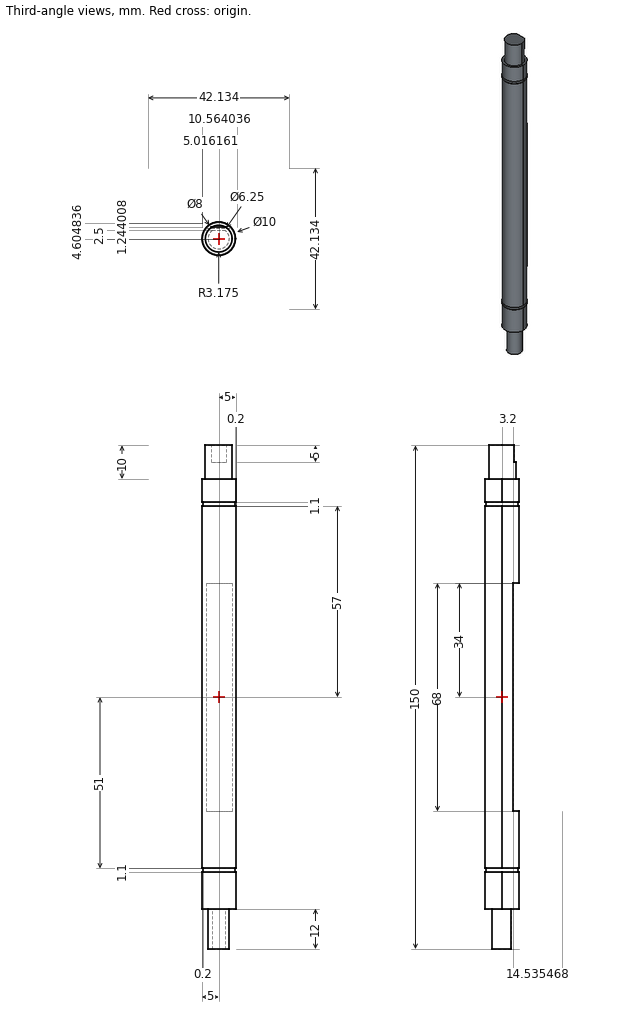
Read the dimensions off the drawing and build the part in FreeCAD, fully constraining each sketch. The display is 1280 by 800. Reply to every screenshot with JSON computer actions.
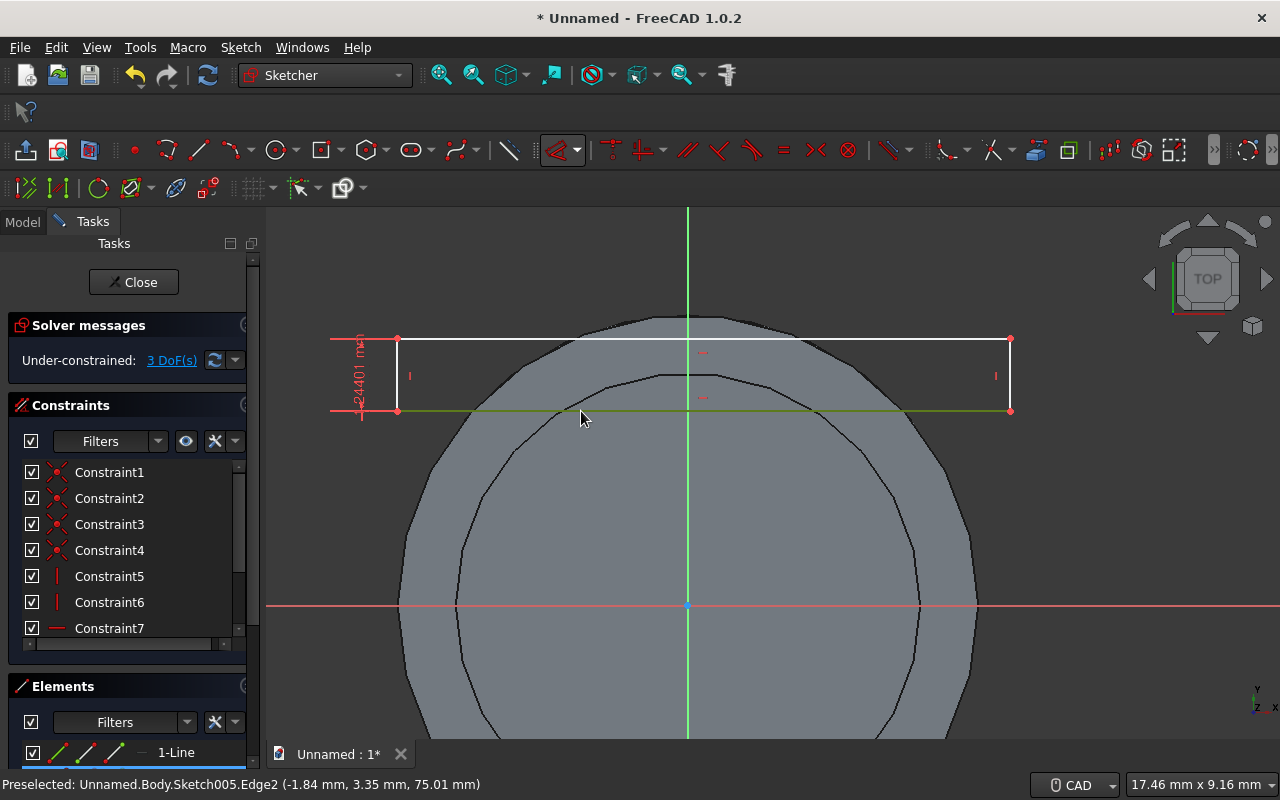
{"action": "key", "text": "l"}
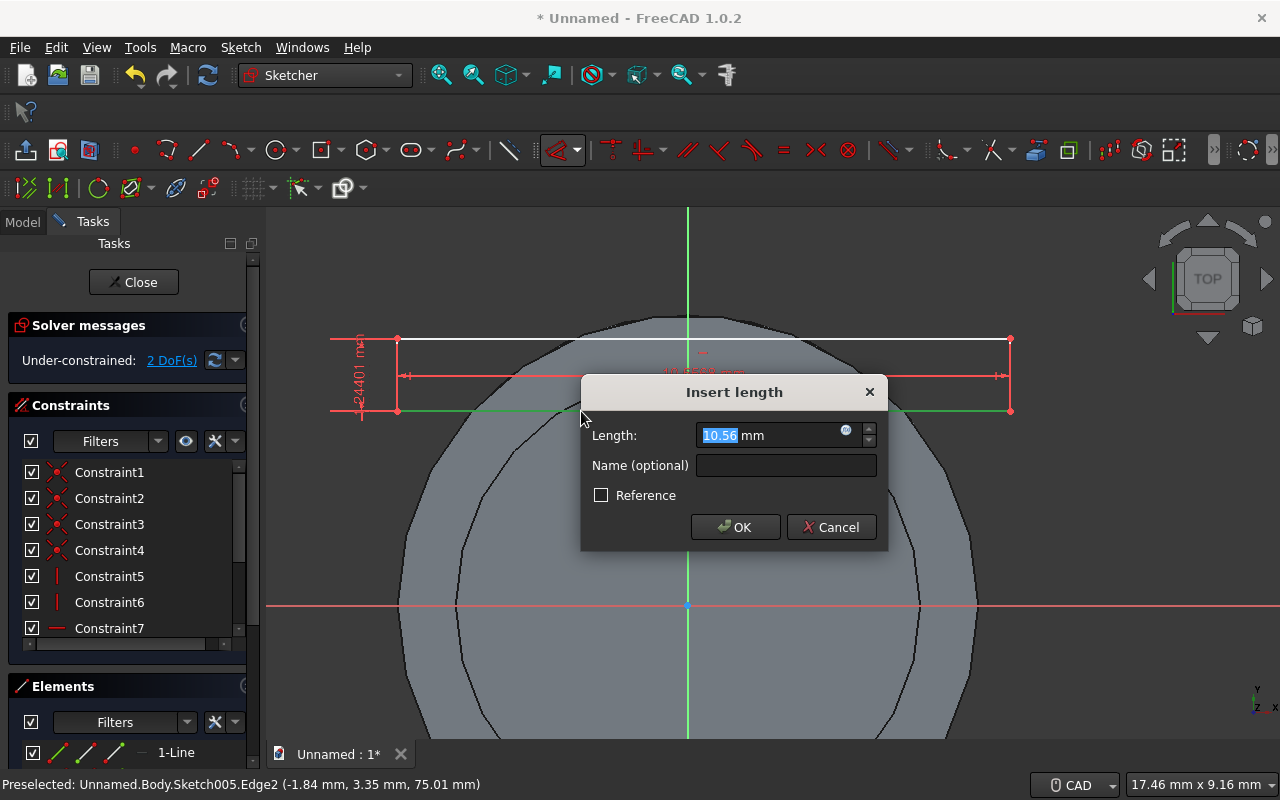
{"action": "type", "text": "10.564036"}
{"action": "key", "text": "Return"}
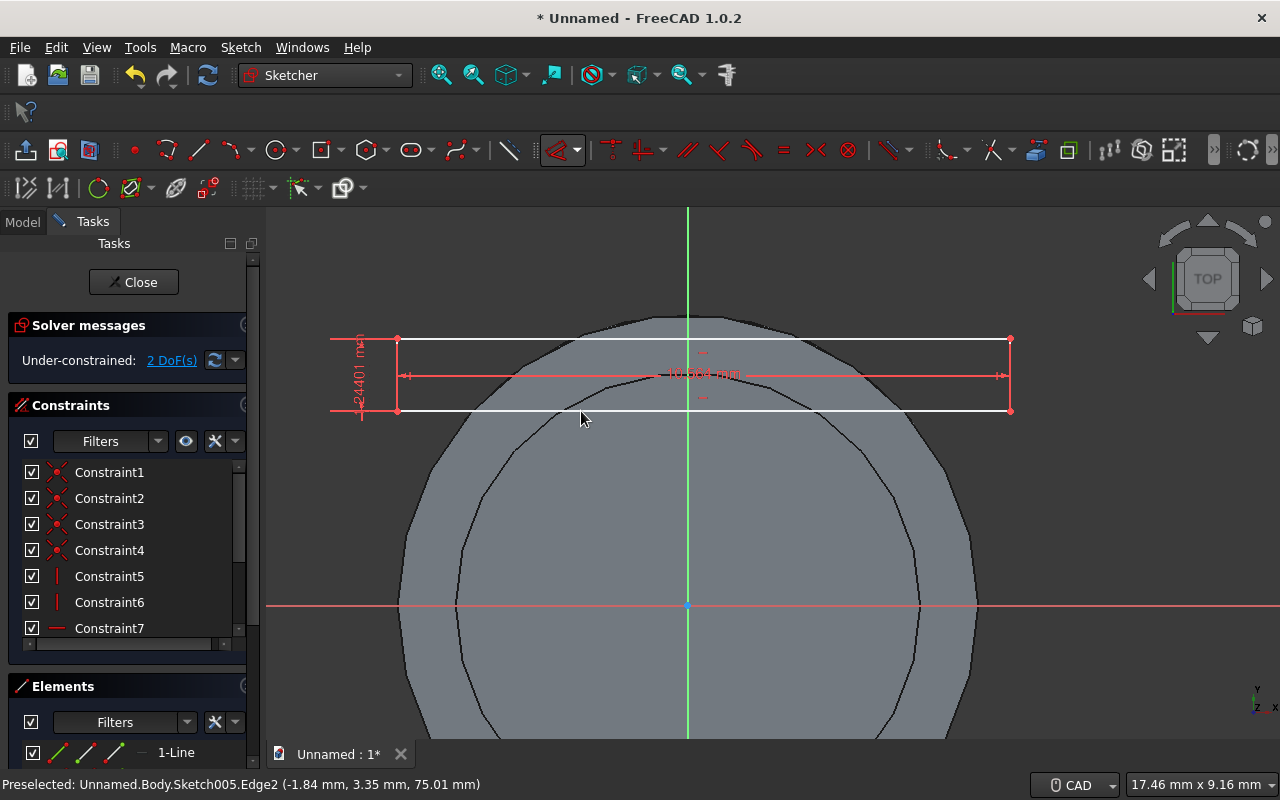
{"action": "left_click", "coordinate": [397, 339]}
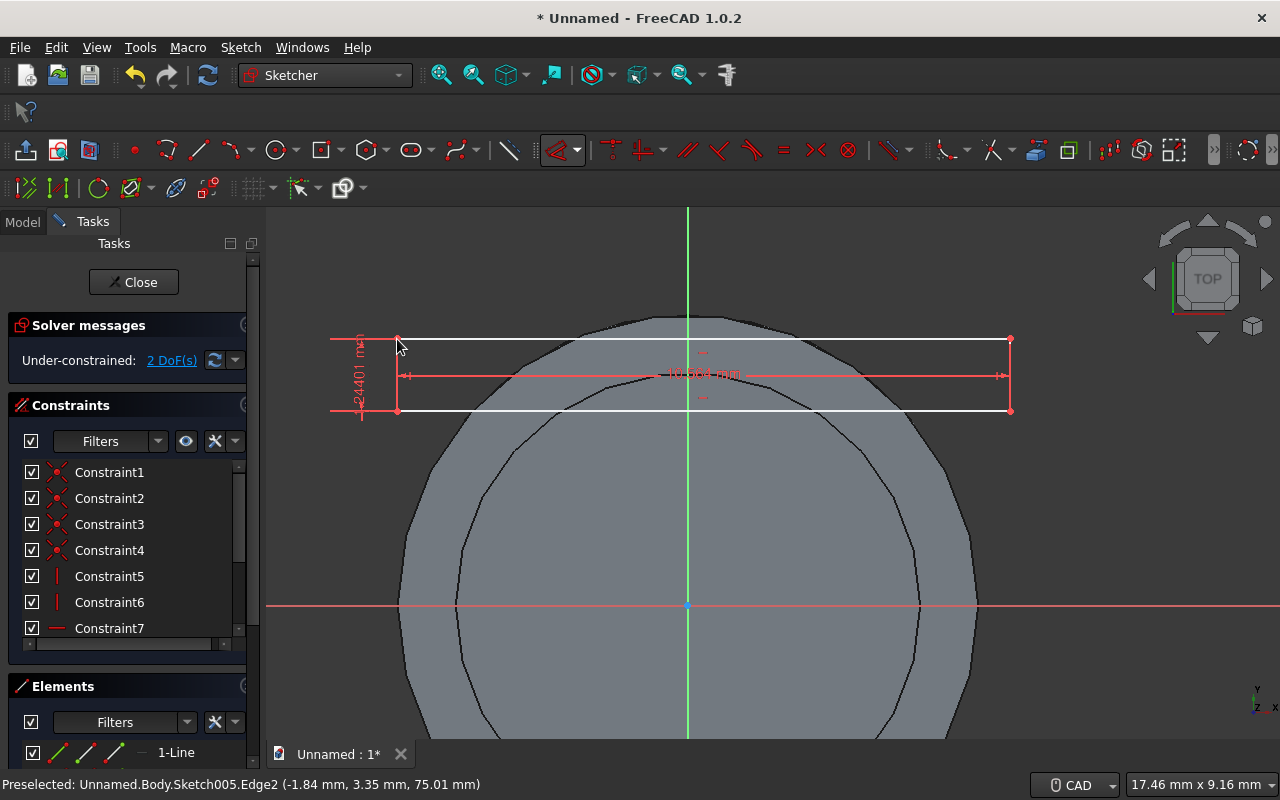
{"action": "left_click", "coordinate": [580, 150]}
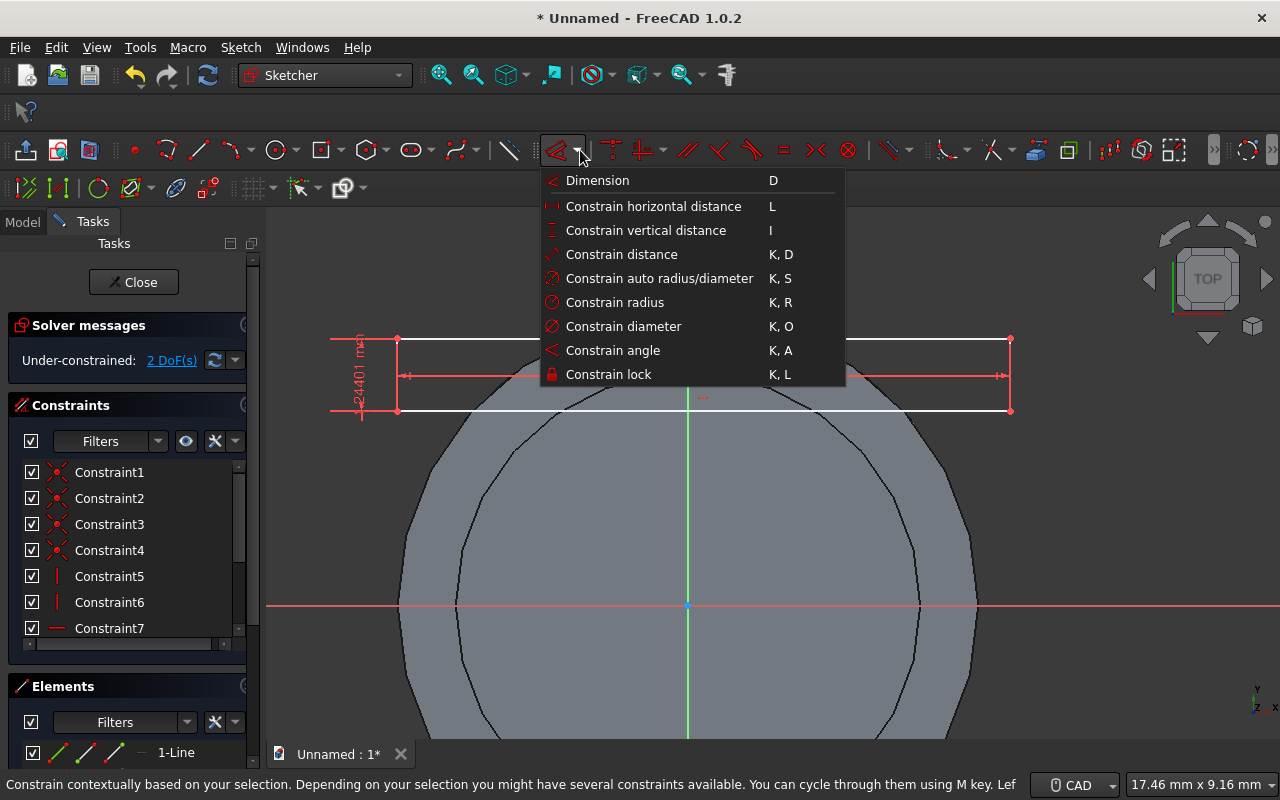
{"action": "left_click", "coordinate": [693, 206]}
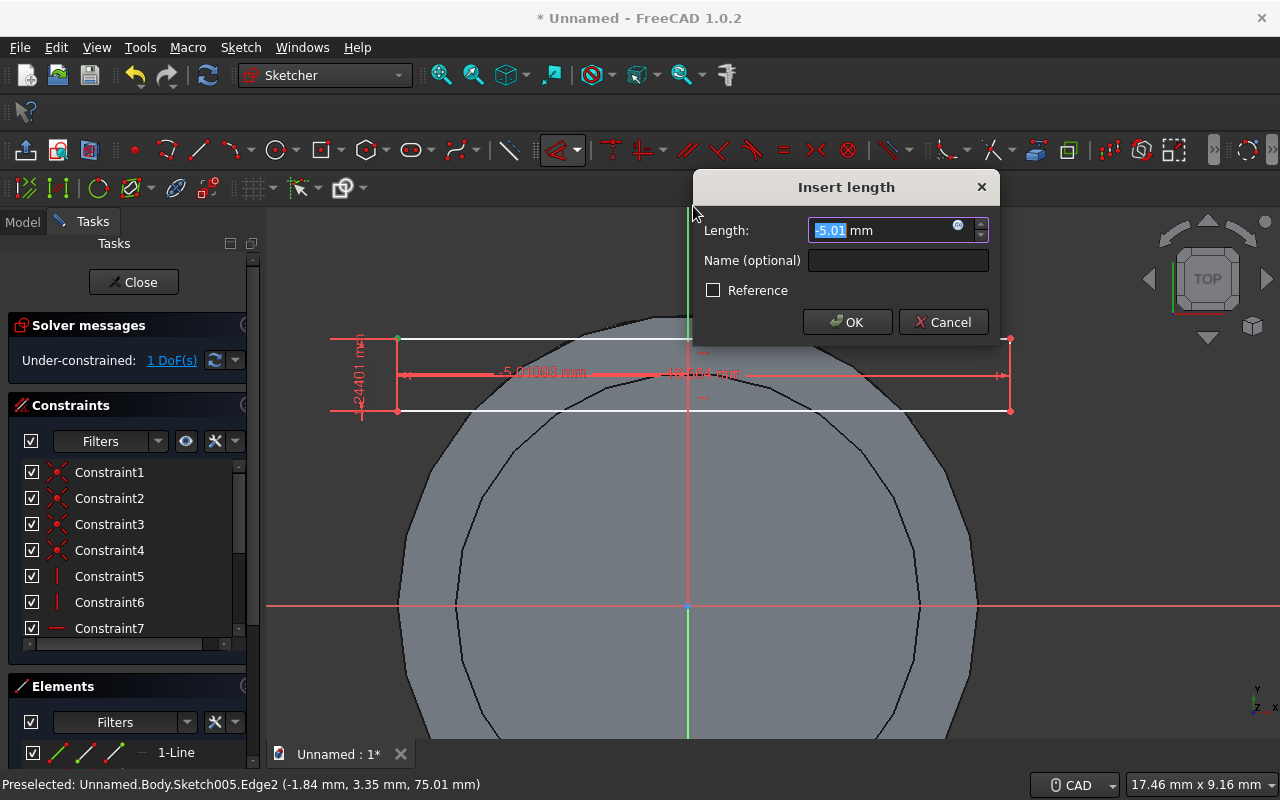
{"action": "type", "text": "-5.016161"}
{"action": "key", "text": "Return"}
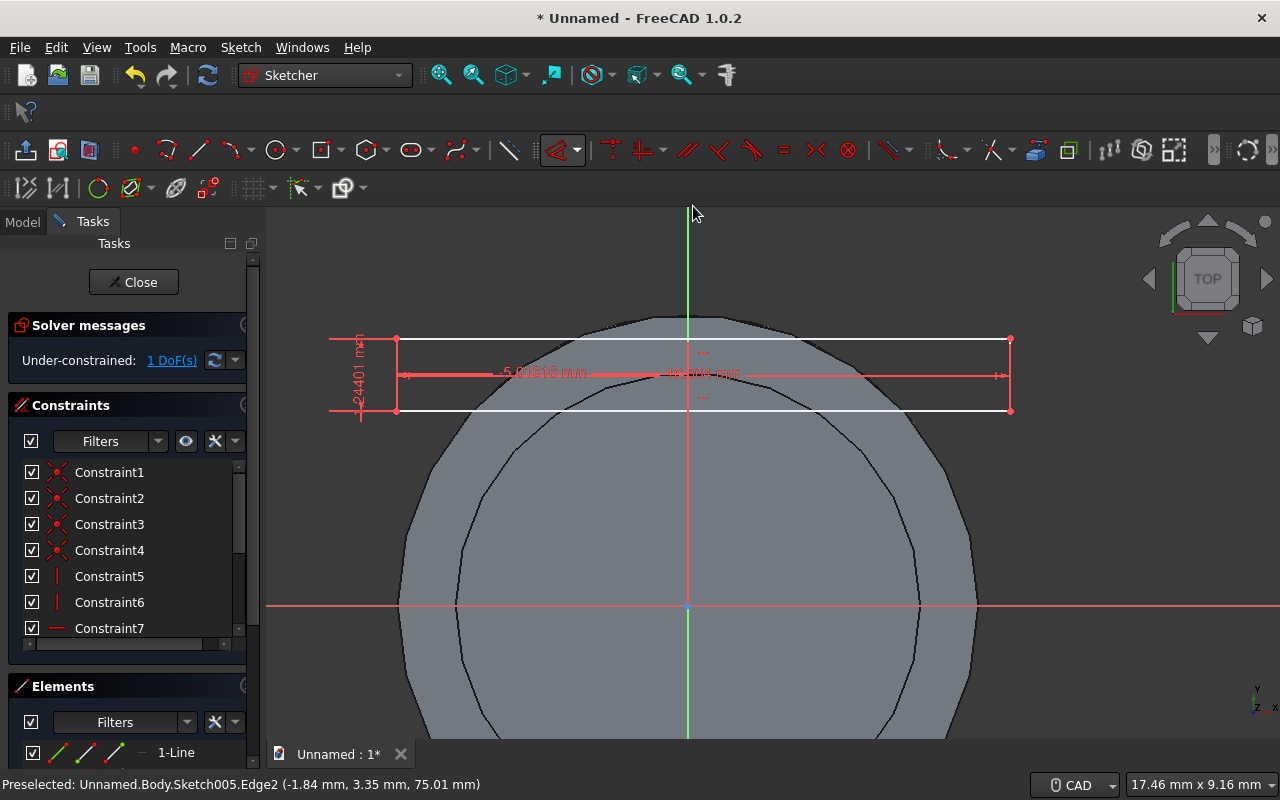
{"action": "left_click", "coordinate": [397, 339]}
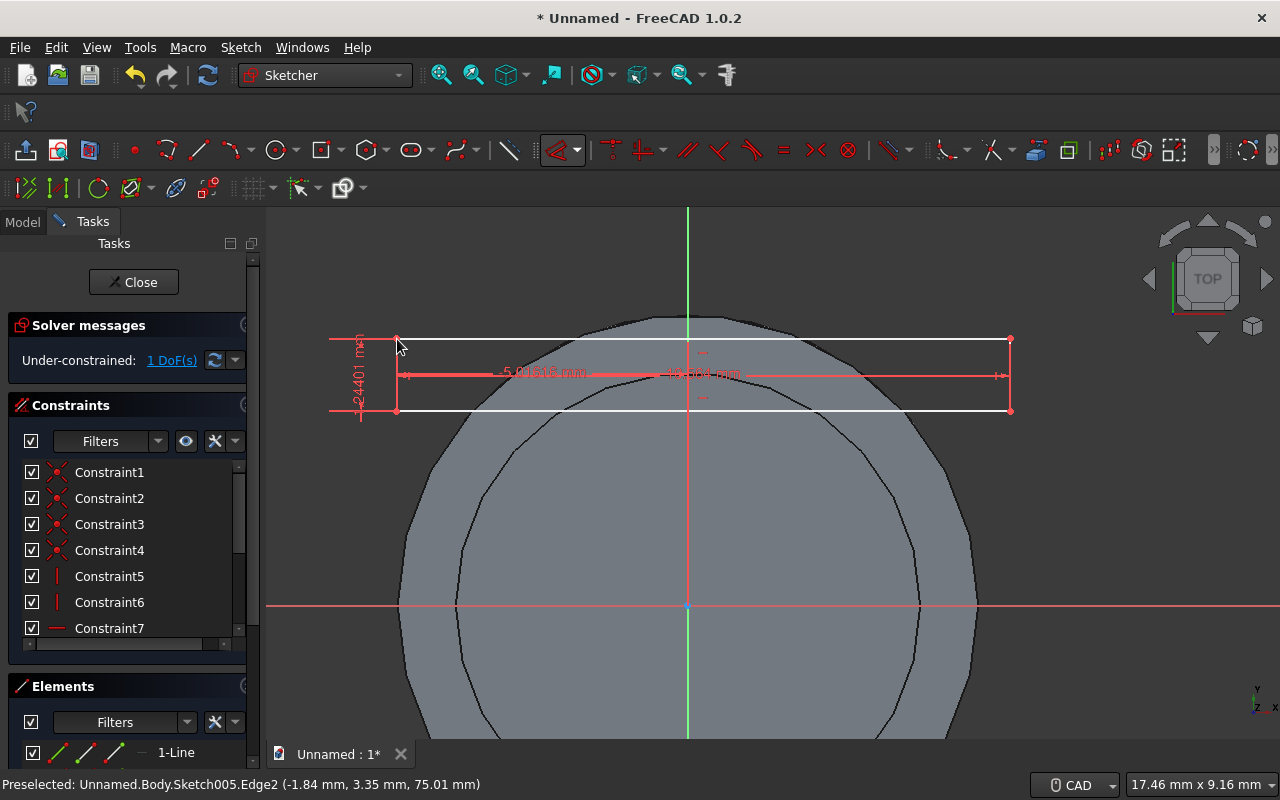
{"action": "left_click", "coordinate": [580, 150]}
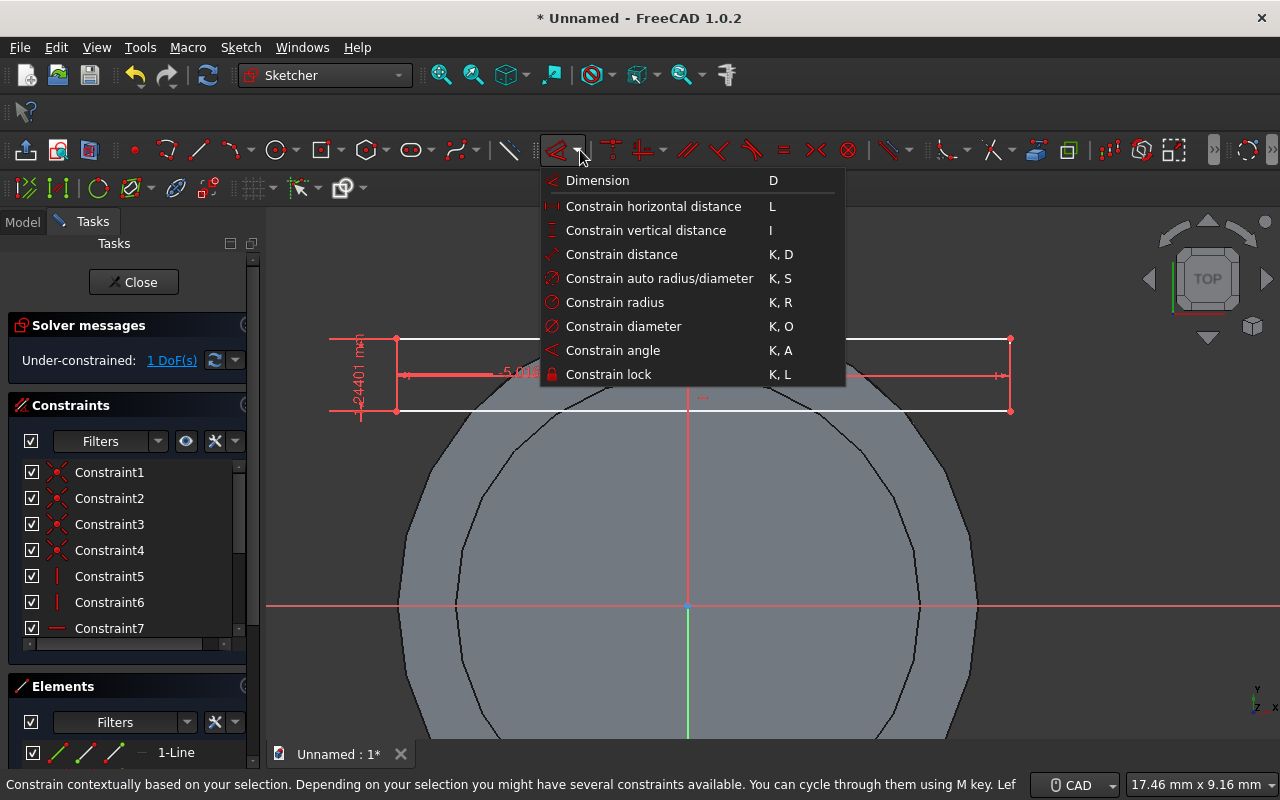
{"action": "left_click", "coordinate": [693, 230]}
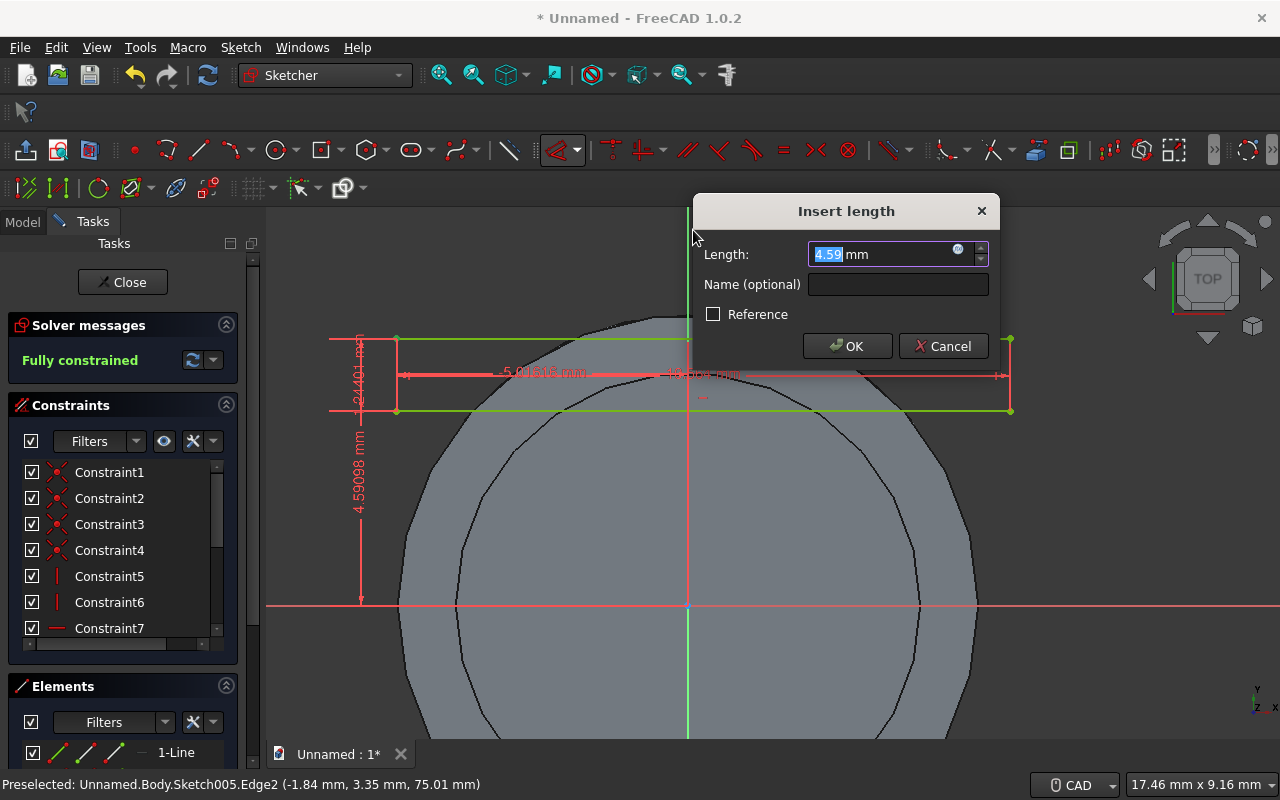
{"action": "type", "text": "4.604836"}
{"action": "key", "text": "Return"}